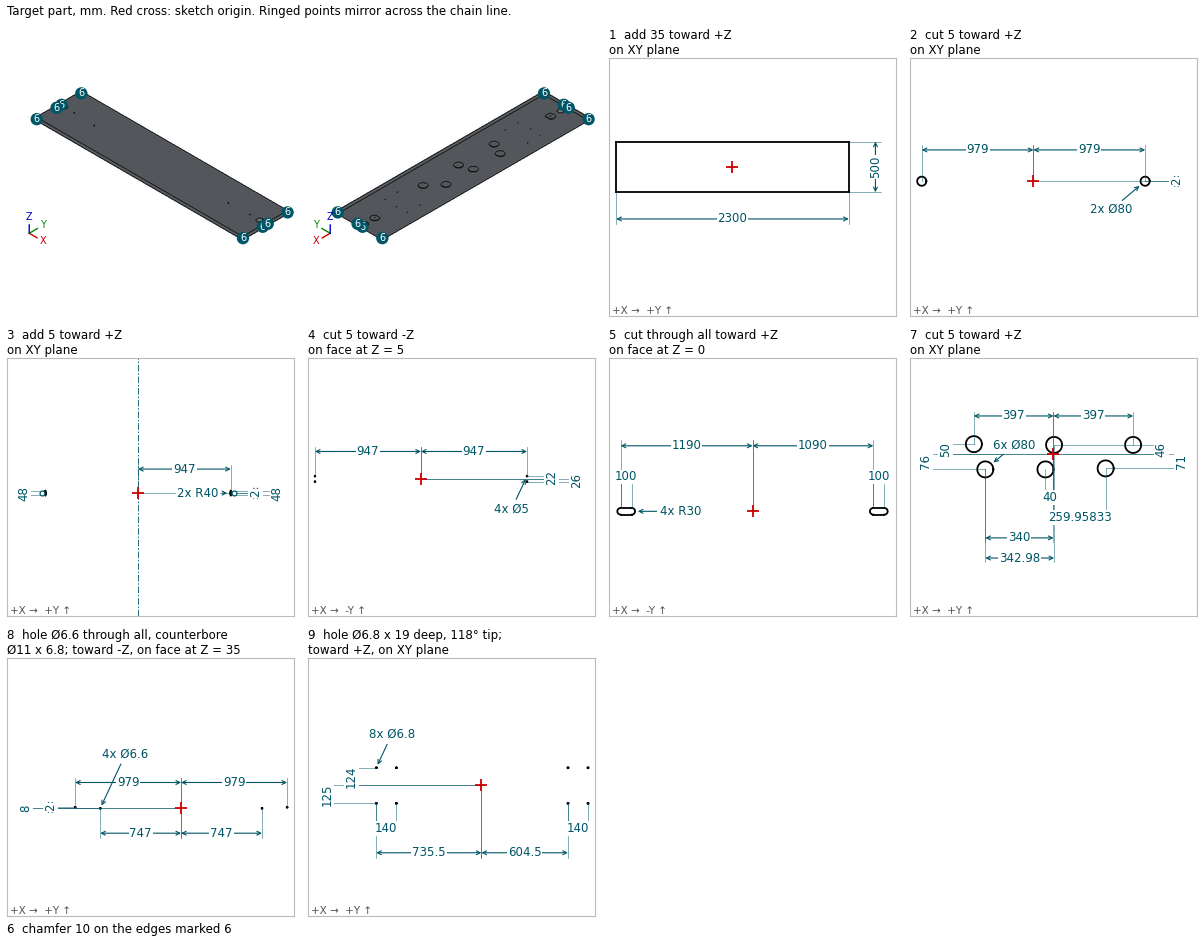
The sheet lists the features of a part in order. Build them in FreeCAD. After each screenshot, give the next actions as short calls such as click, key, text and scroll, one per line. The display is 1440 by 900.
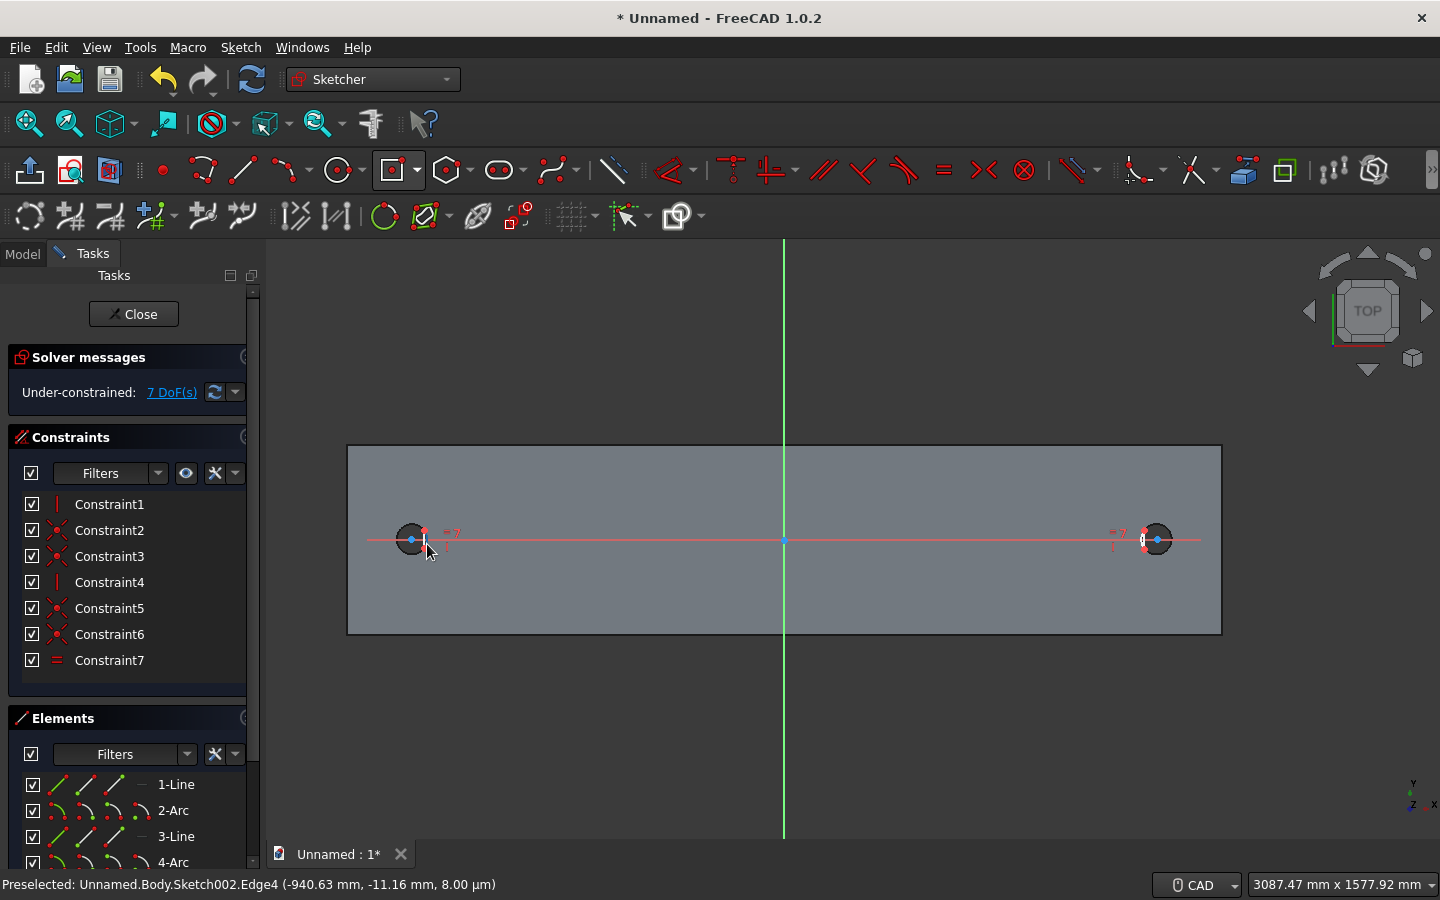
click(1157, 540)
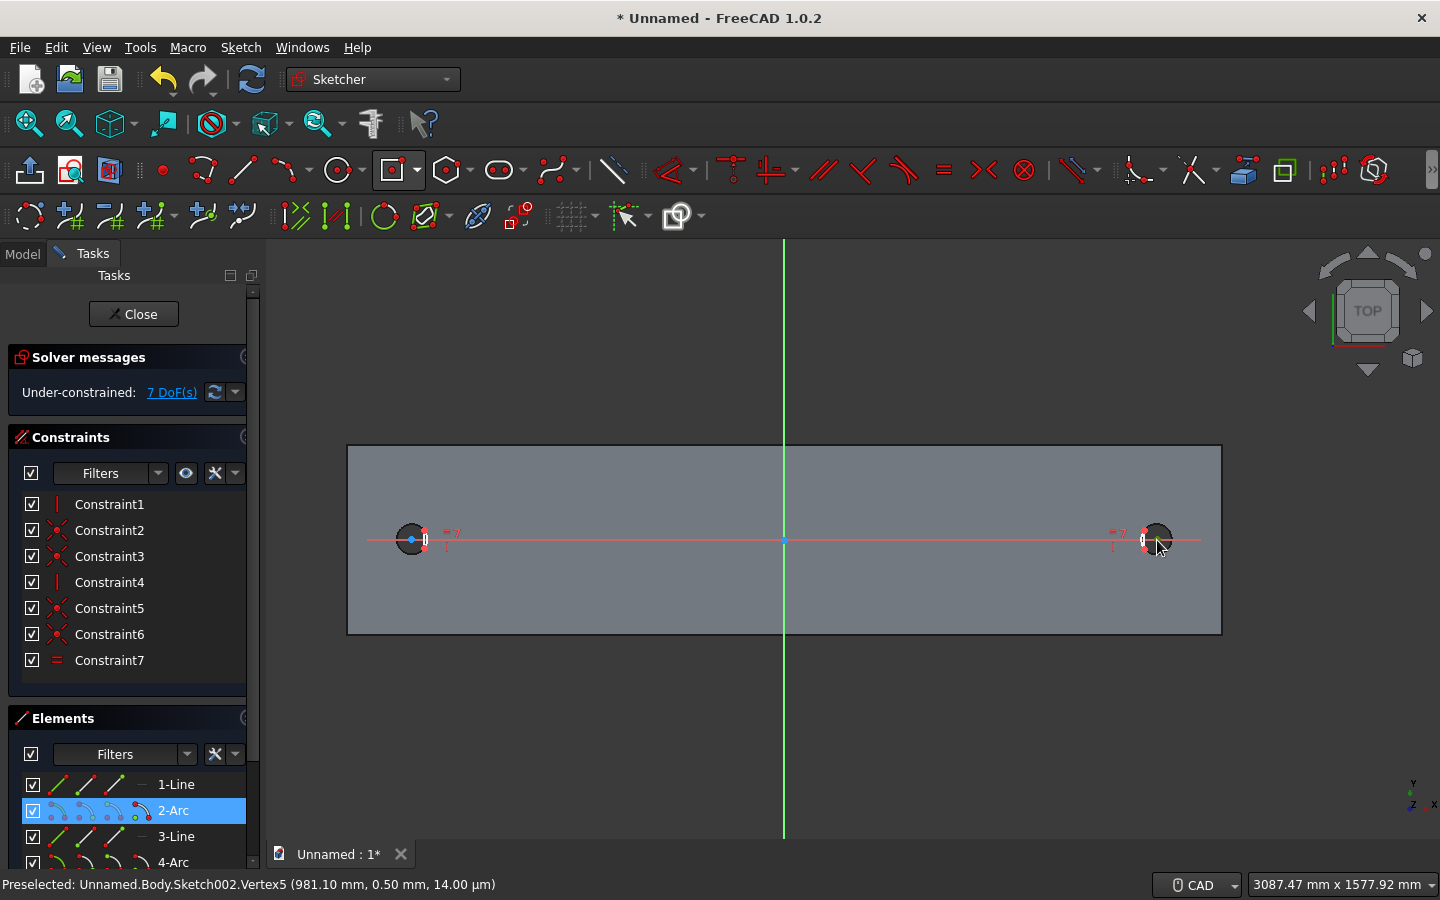
click(411, 540)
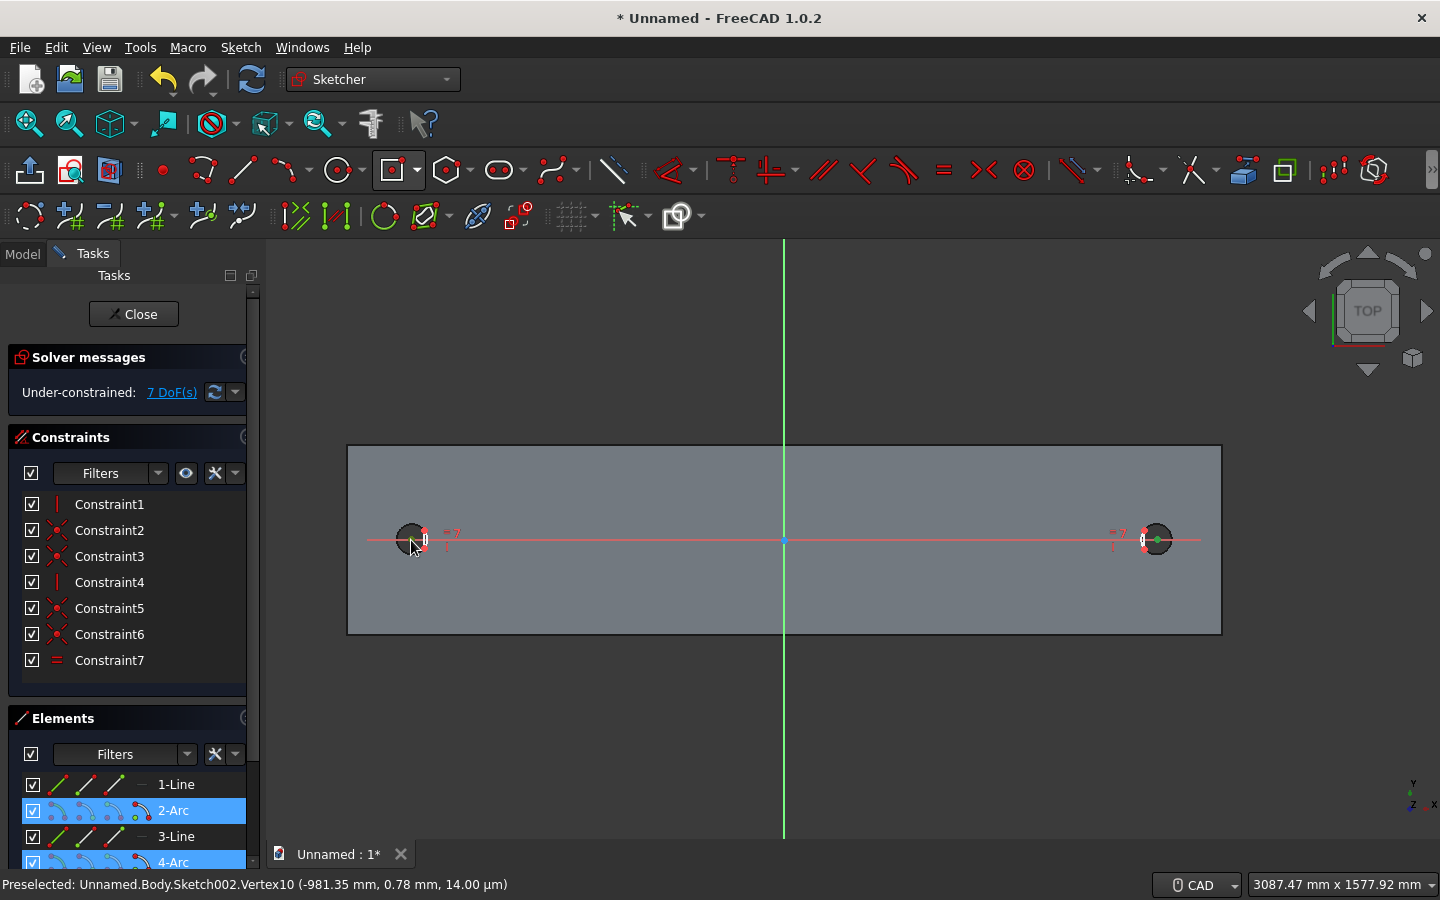
click(784, 772)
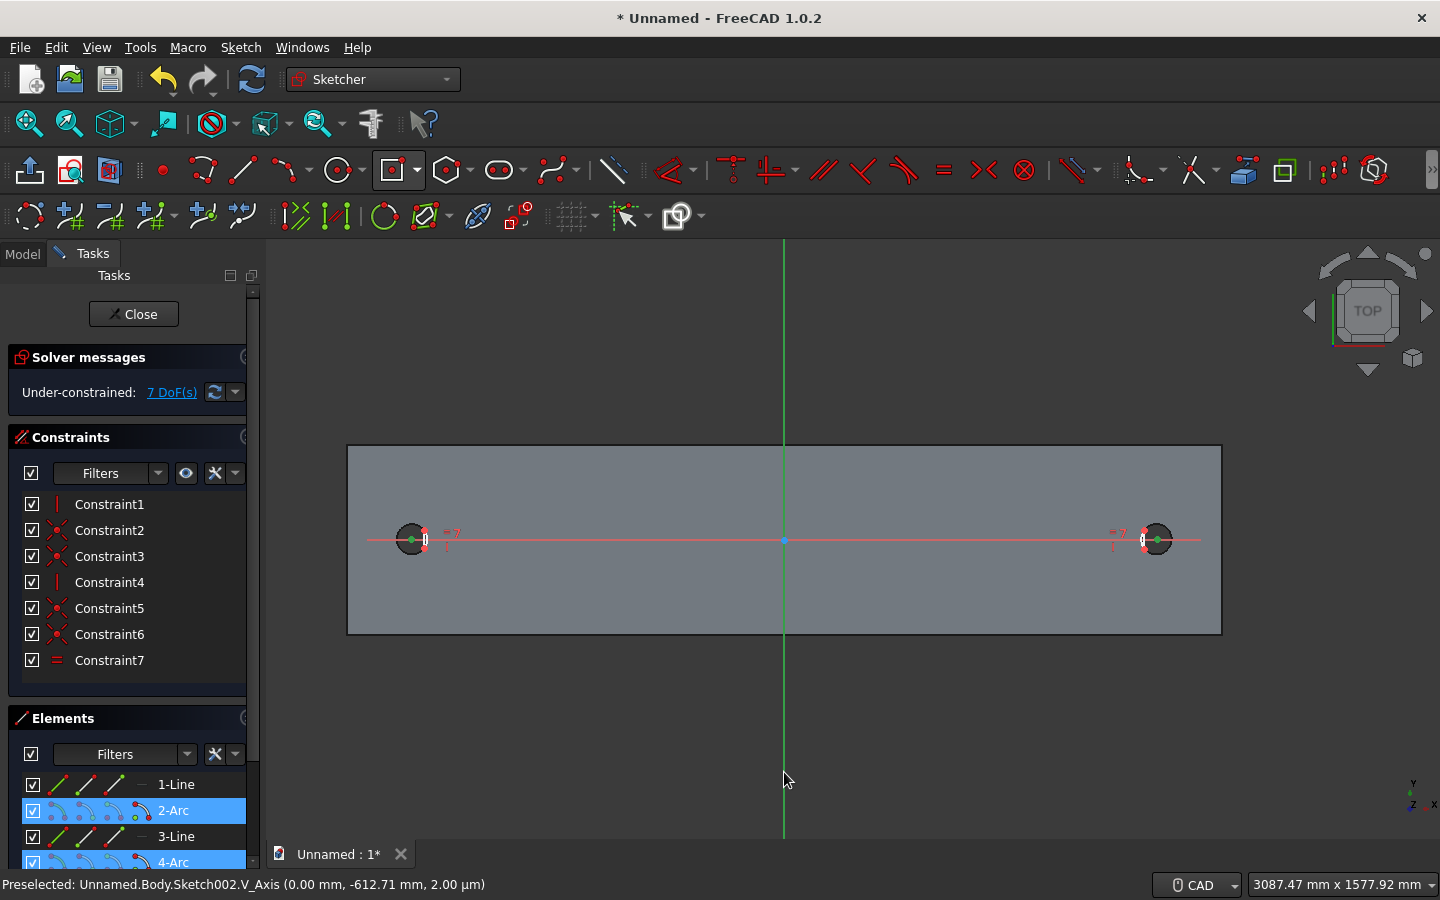
click(984, 170)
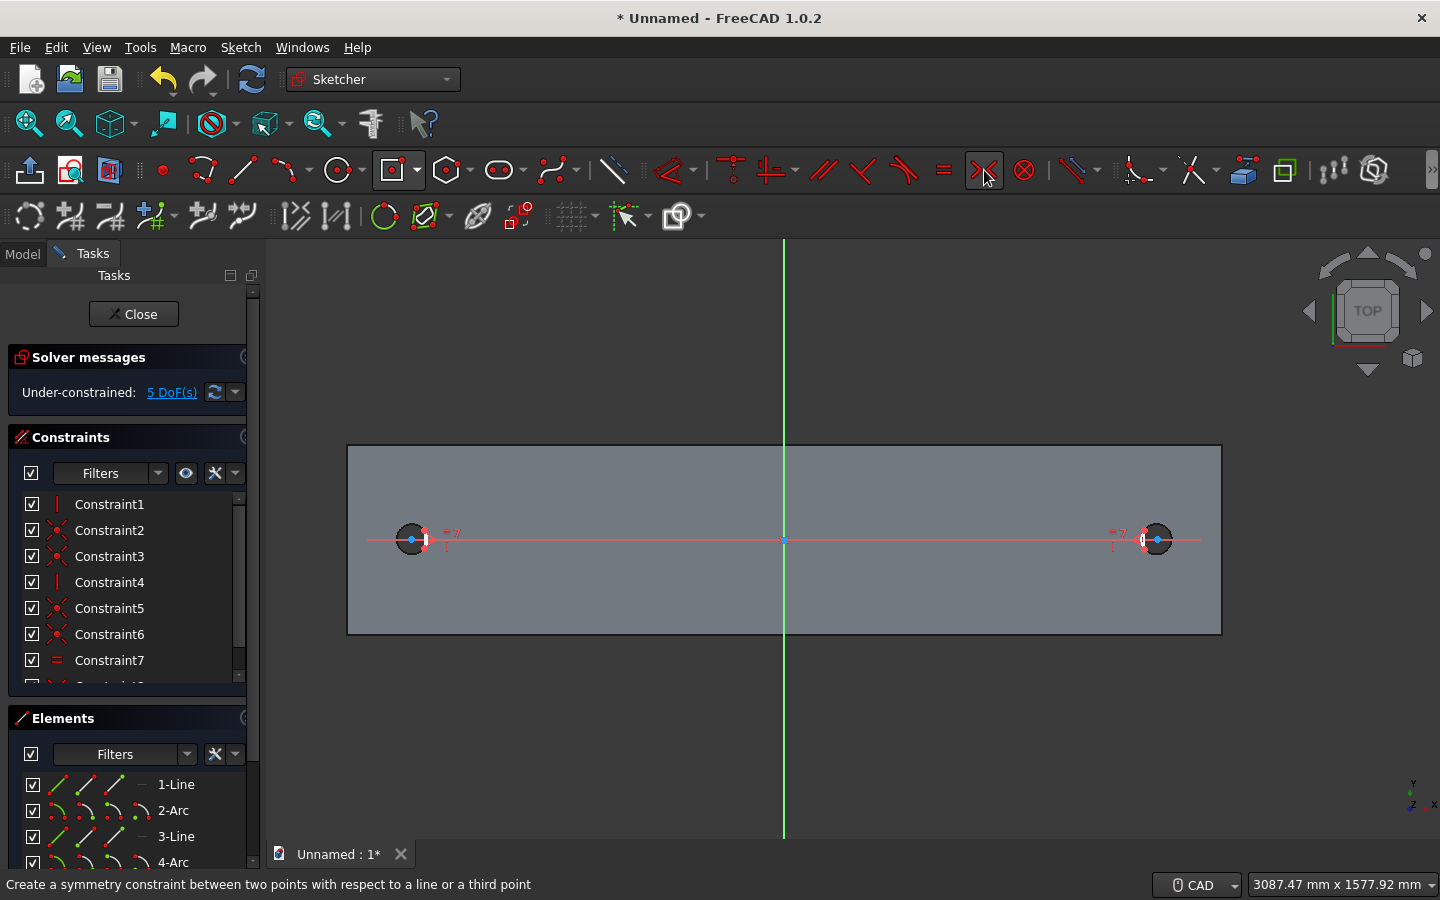
click(668, 170)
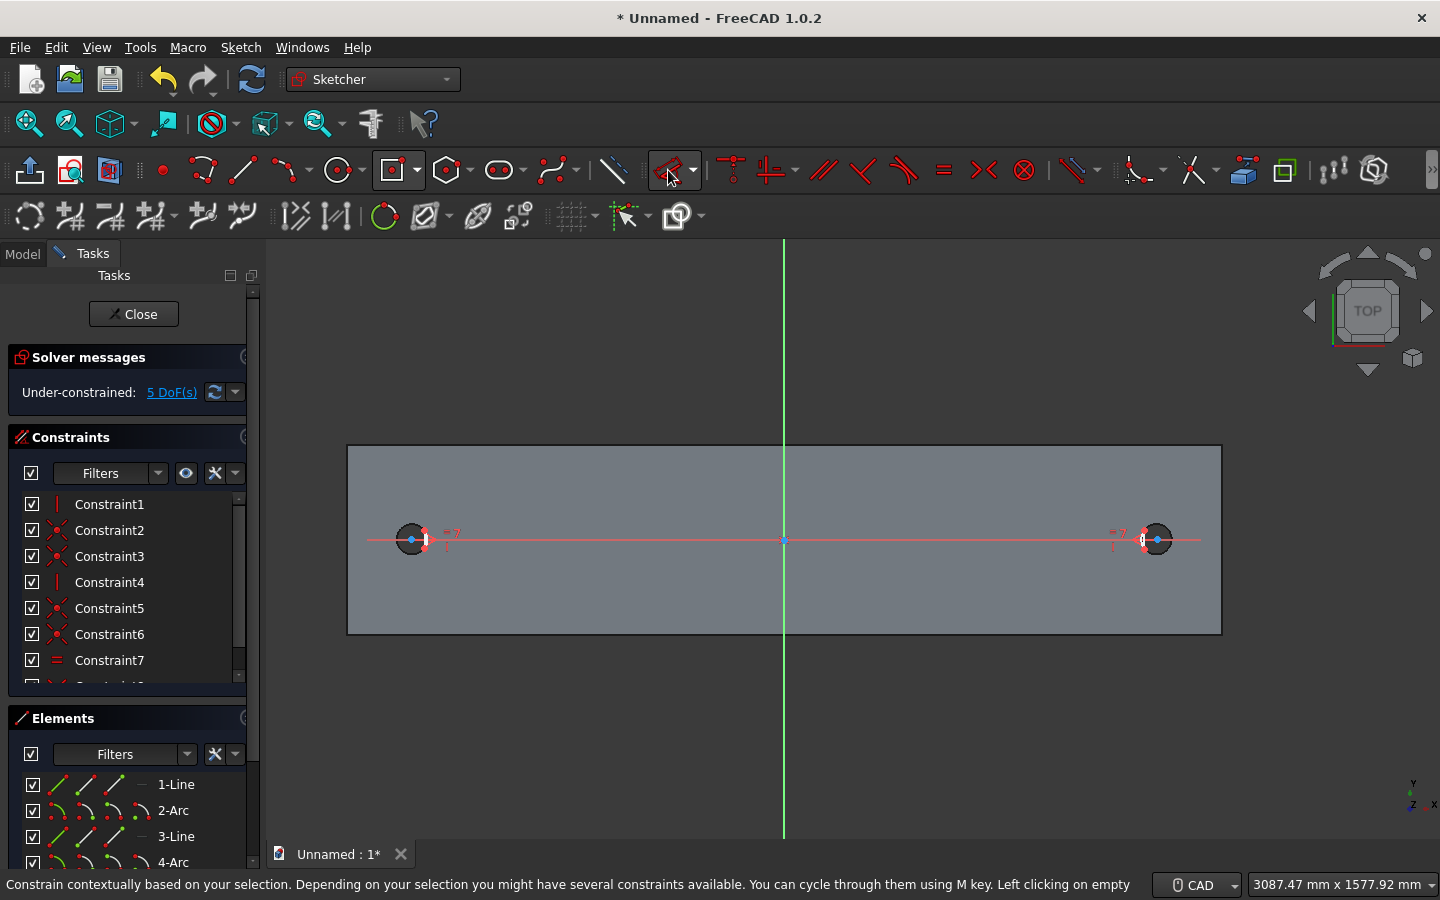
scroll(1141, 540, up, 8)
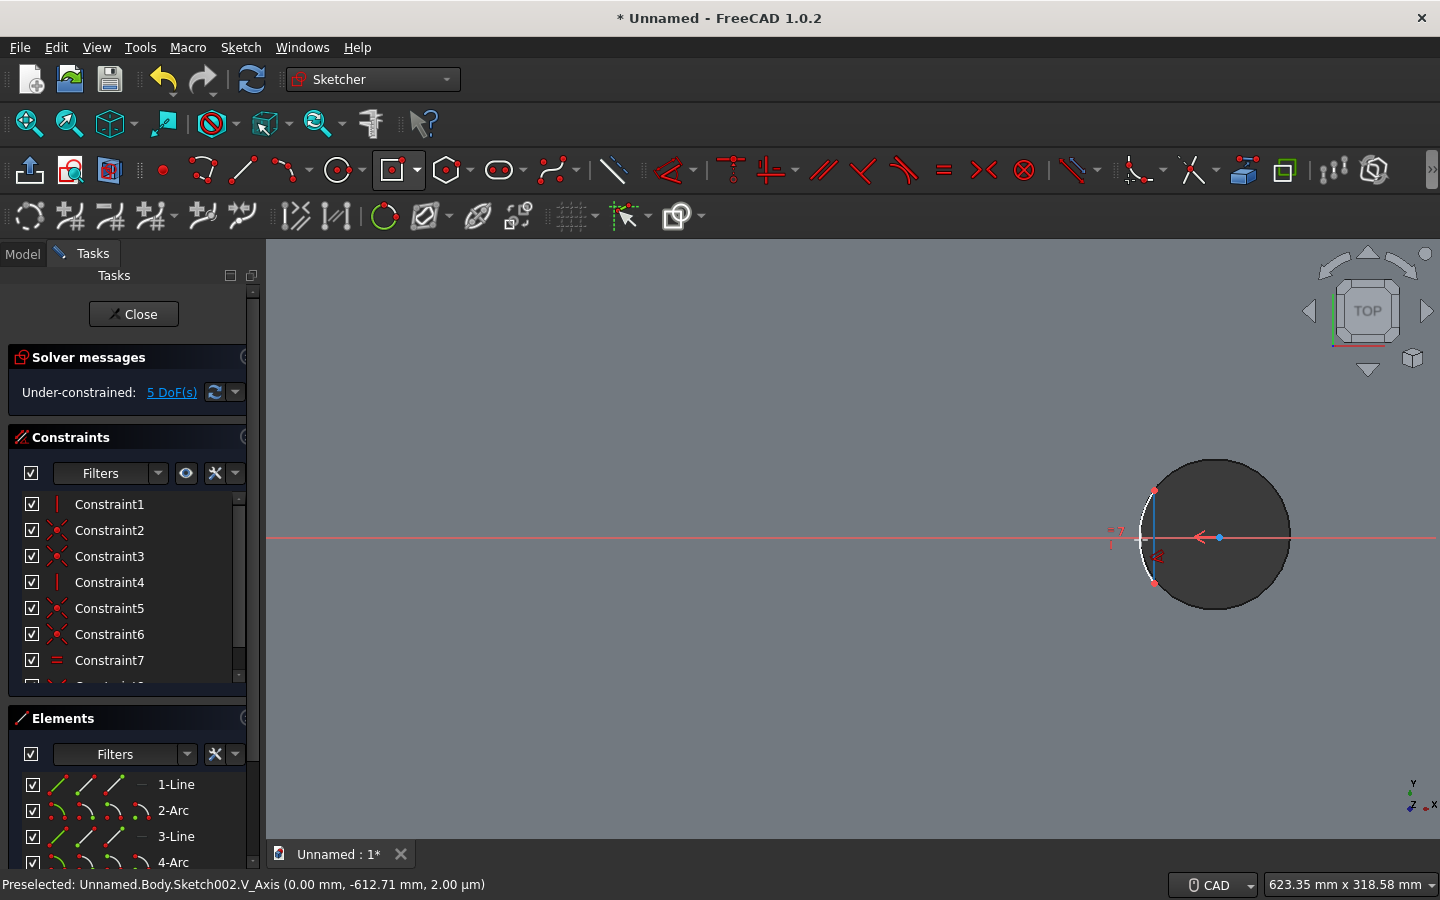
click(1140, 537)
click(1122, 484)